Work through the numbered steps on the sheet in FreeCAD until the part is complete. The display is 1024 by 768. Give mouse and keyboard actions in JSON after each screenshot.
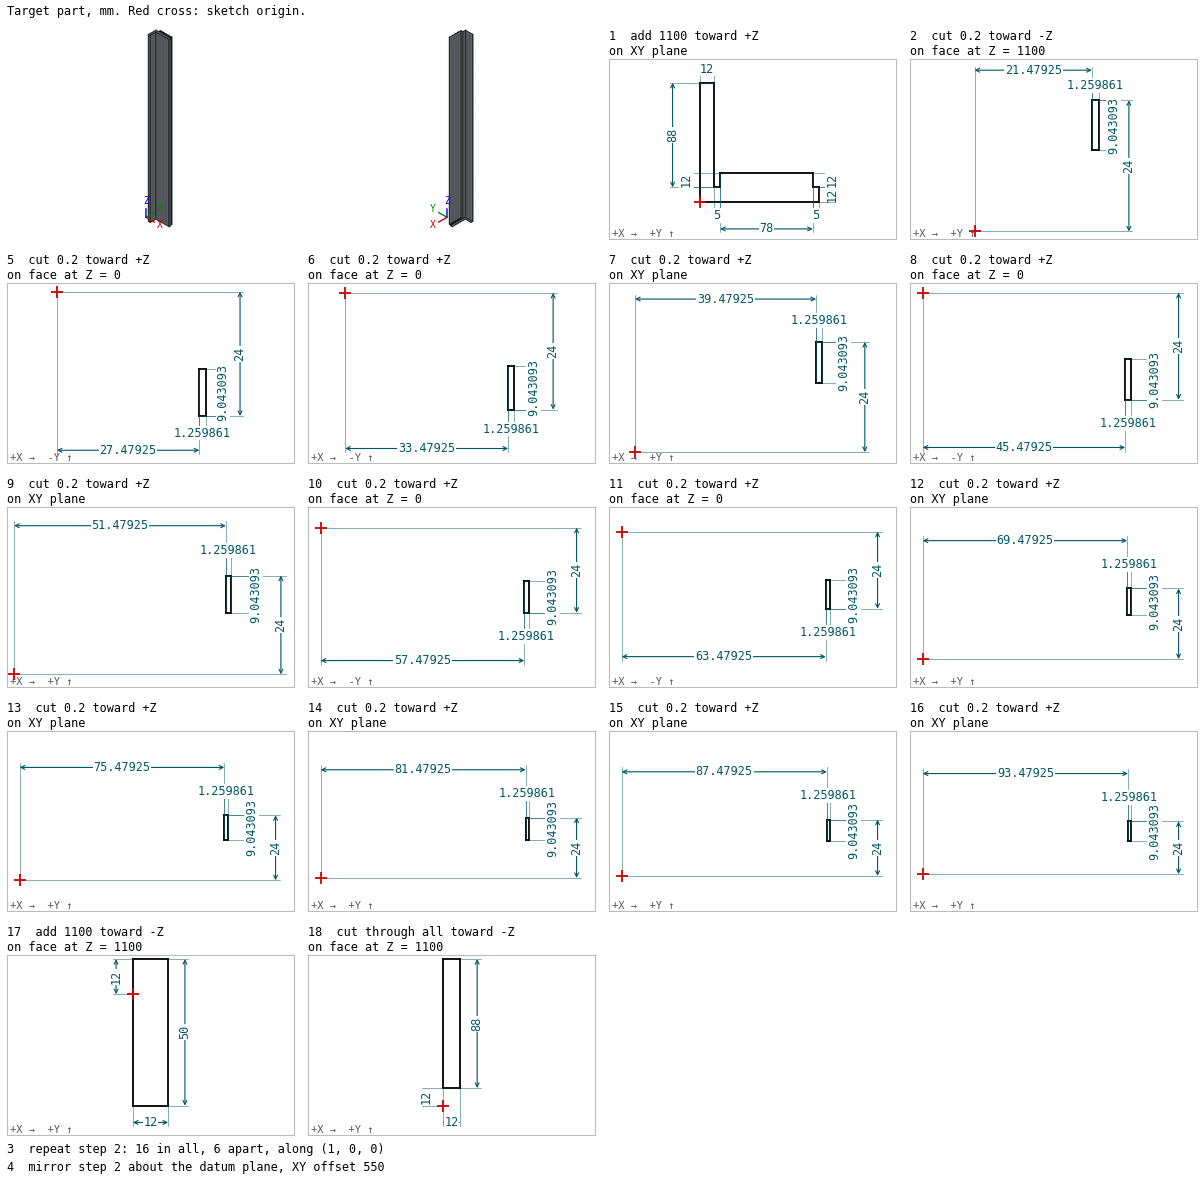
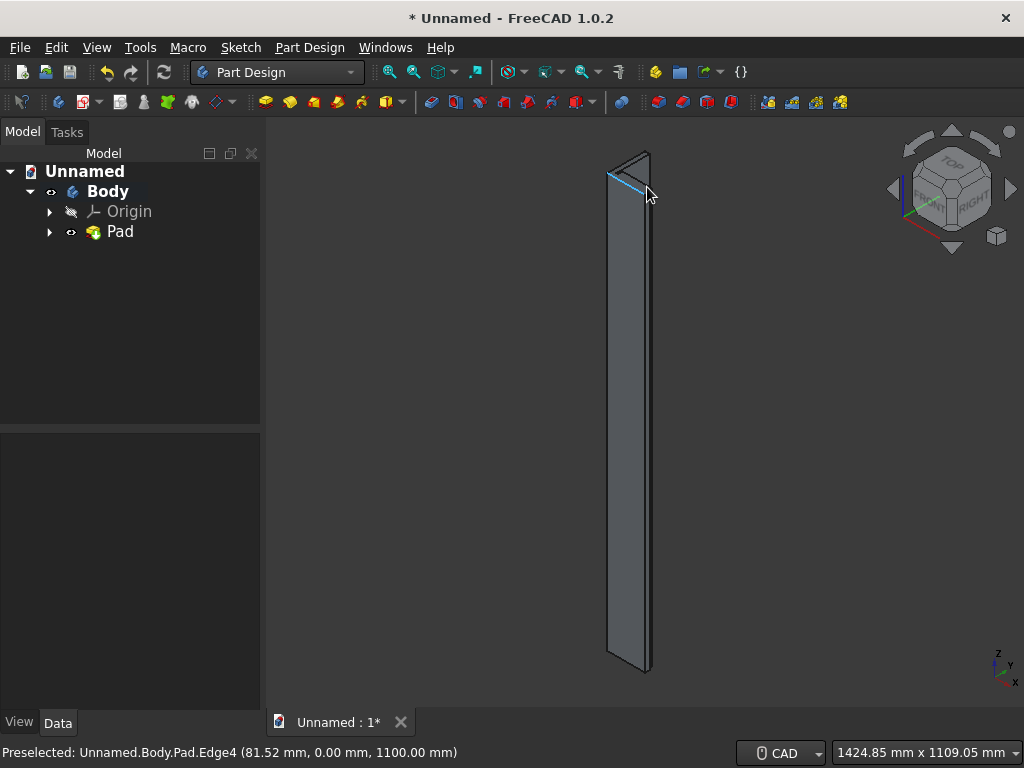
{"action": "scroll", "coordinate": [640, 188], "scroll_direction": "up", "scroll_amount": 6}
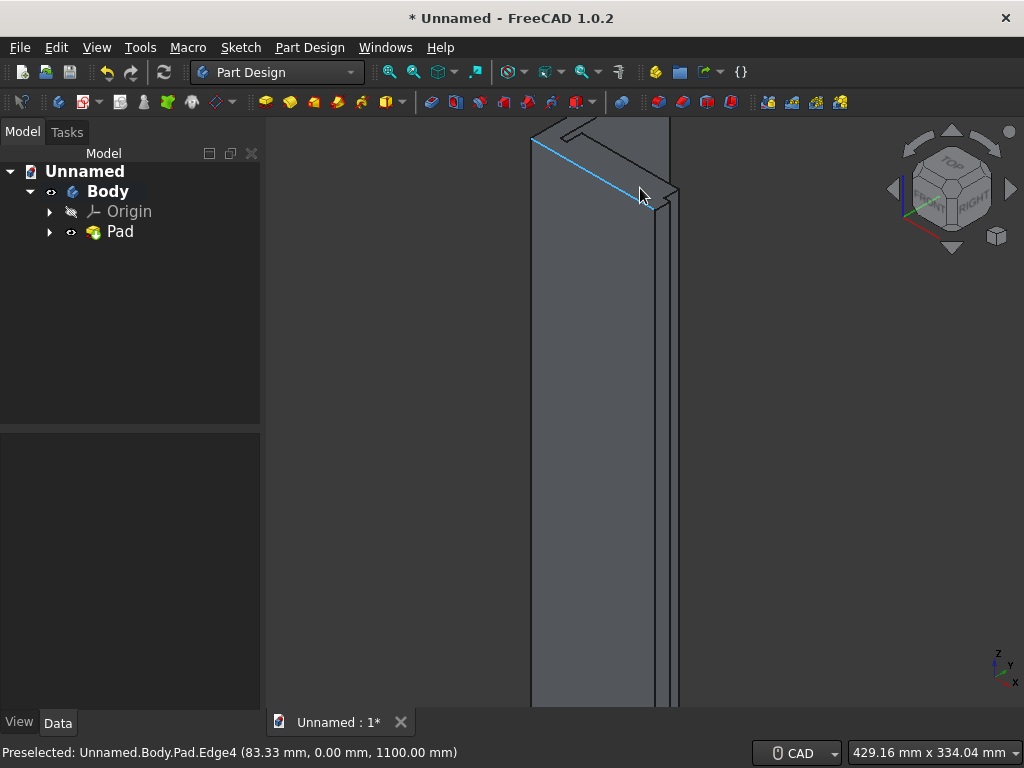
{"action": "left_click", "coordinate": [620, 178]}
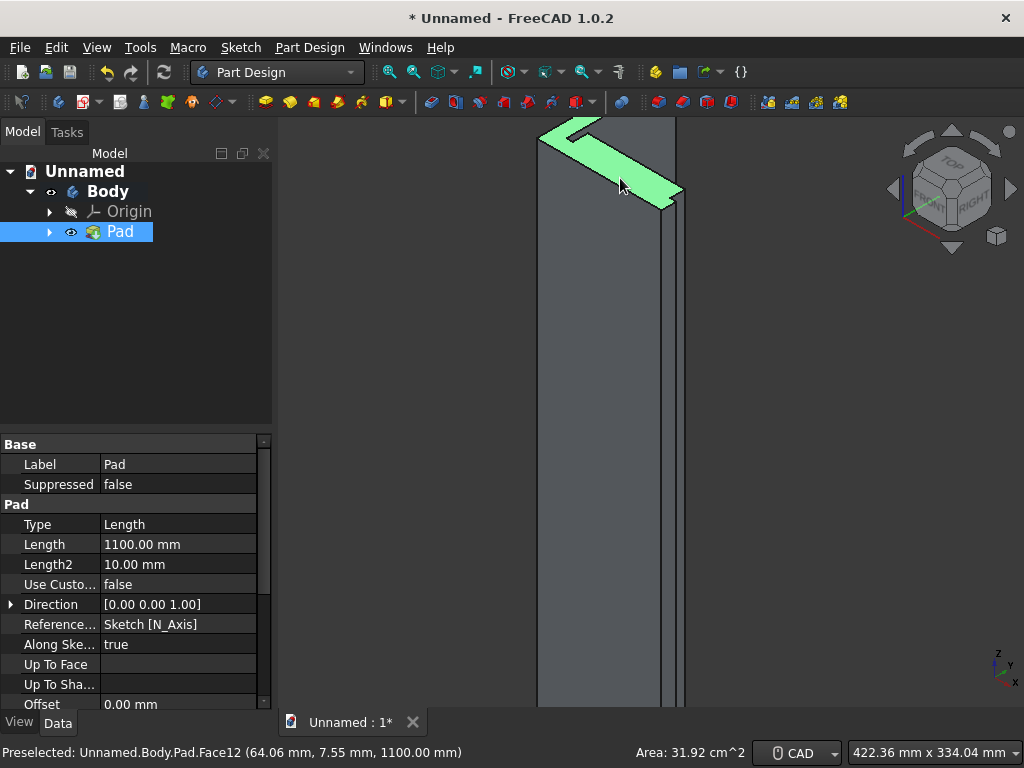
{"action": "left_click", "coordinate": [84, 102]}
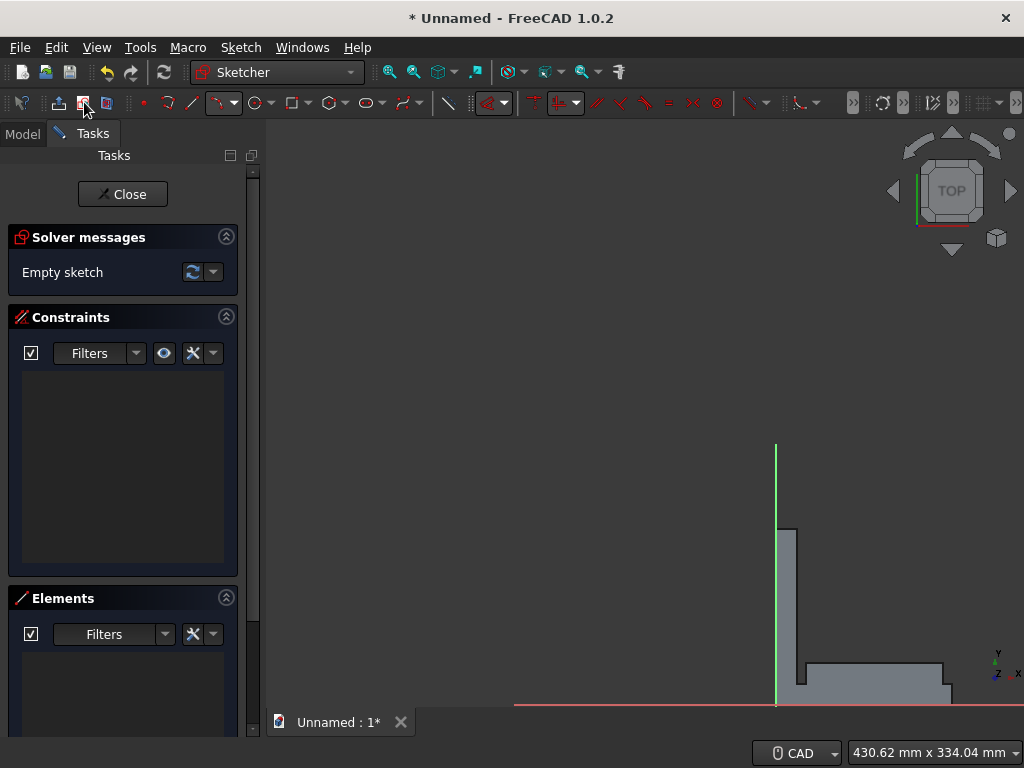
{"action": "scroll", "coordinate": [576, 413], "scroll_direction": "down", "scroll_amount": 5}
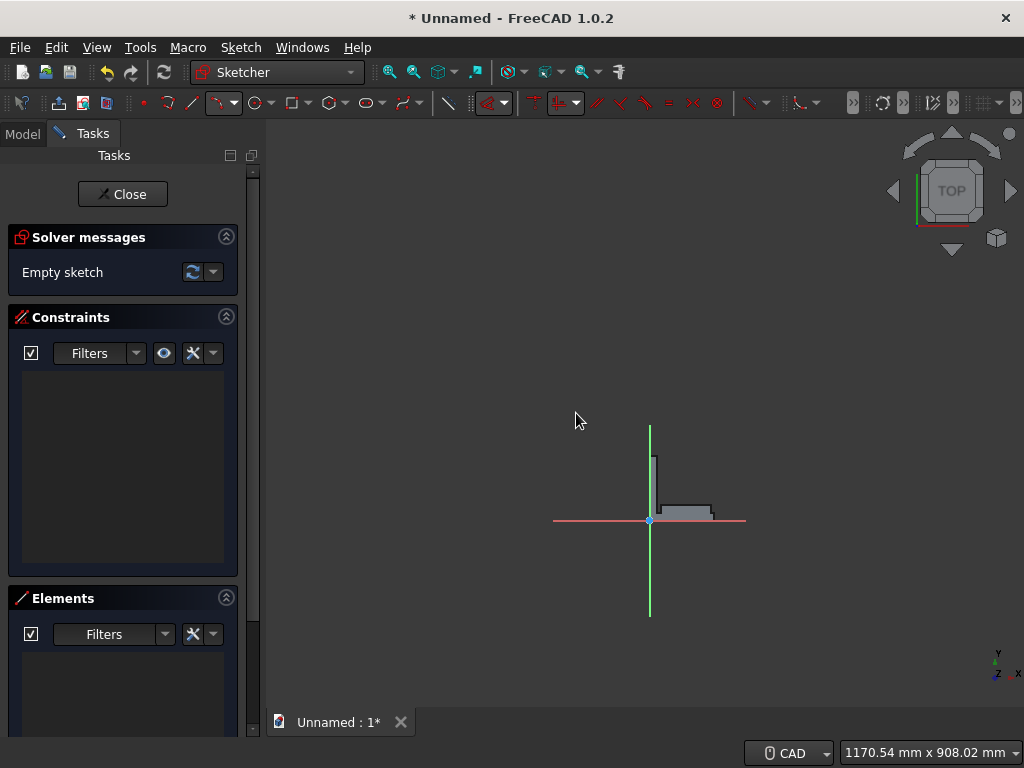
{"action": "scroll", "coordinate": [669, 513], "scroll_direction": "up", "scroll_amount": 15}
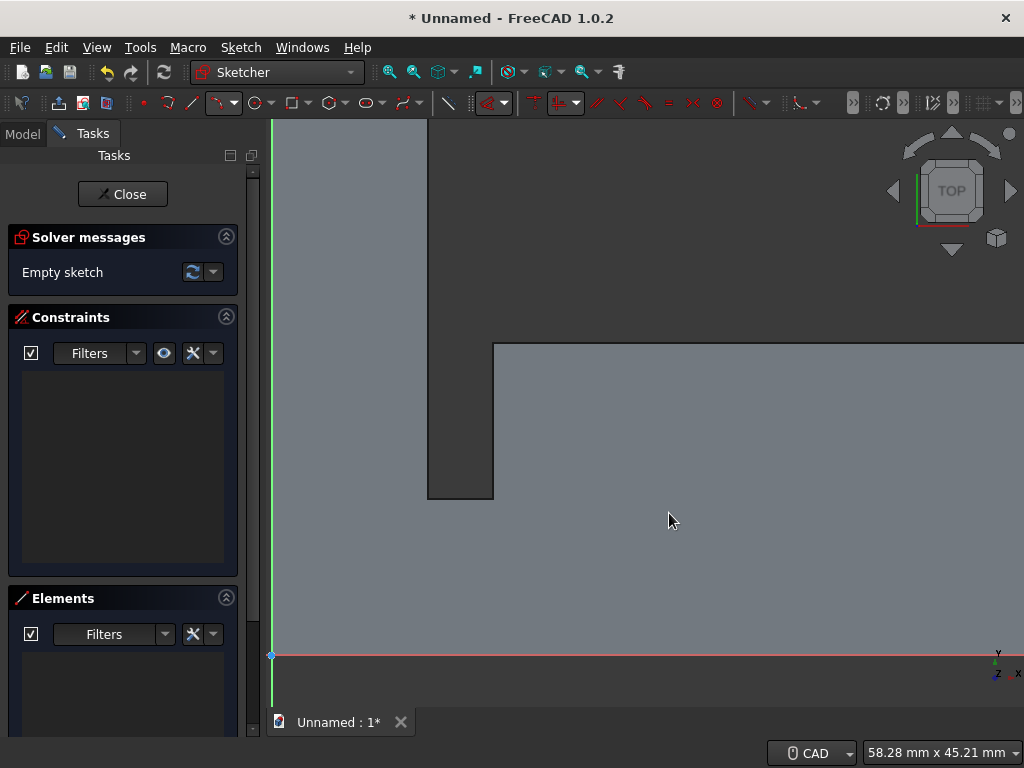
{"action": "scroll", "coordinate": [552, 397], "scroll_direction": "up", "scroll_amount": 6}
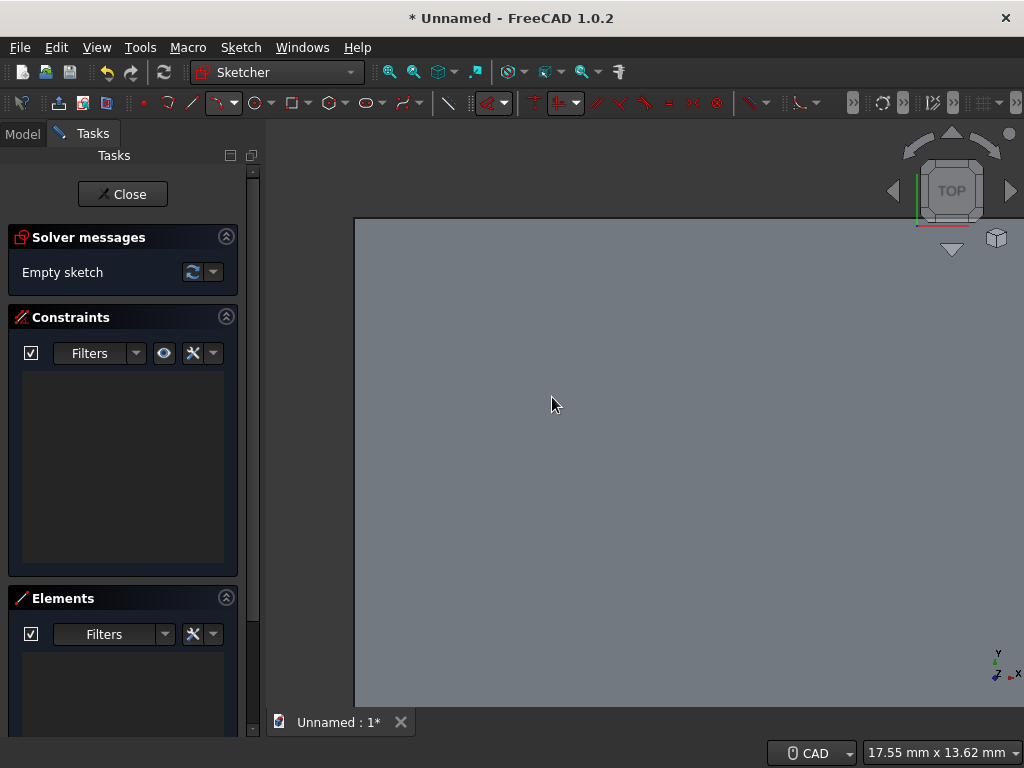
{"action": "left_click", "coordinate": [292, 104]}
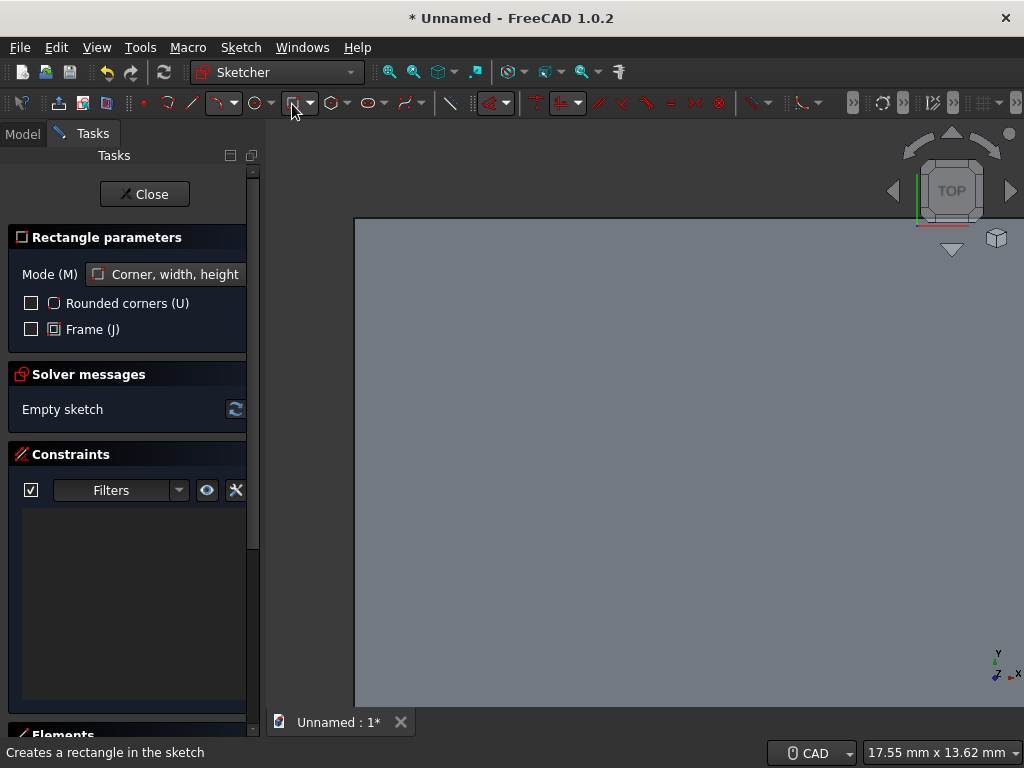
{"action": "left_click", "coordinate": [548, 218]}
{"action": "mouse_move", "coordinate": [602, 608]}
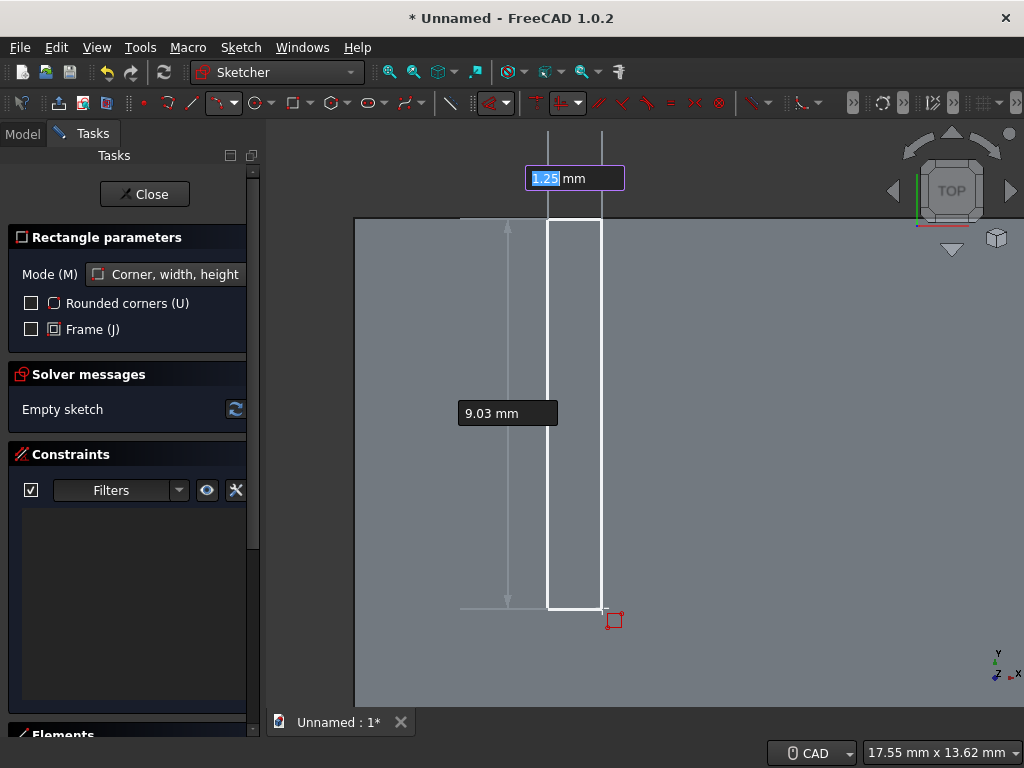
{"action": "type", "text": "1.259861"}
{"action": "key", "text": "Tab"}
{"action": "type", "text": "9.043093"}
{"action": "key", "text": "Return"}
{"action": "key", "text": "Escape"}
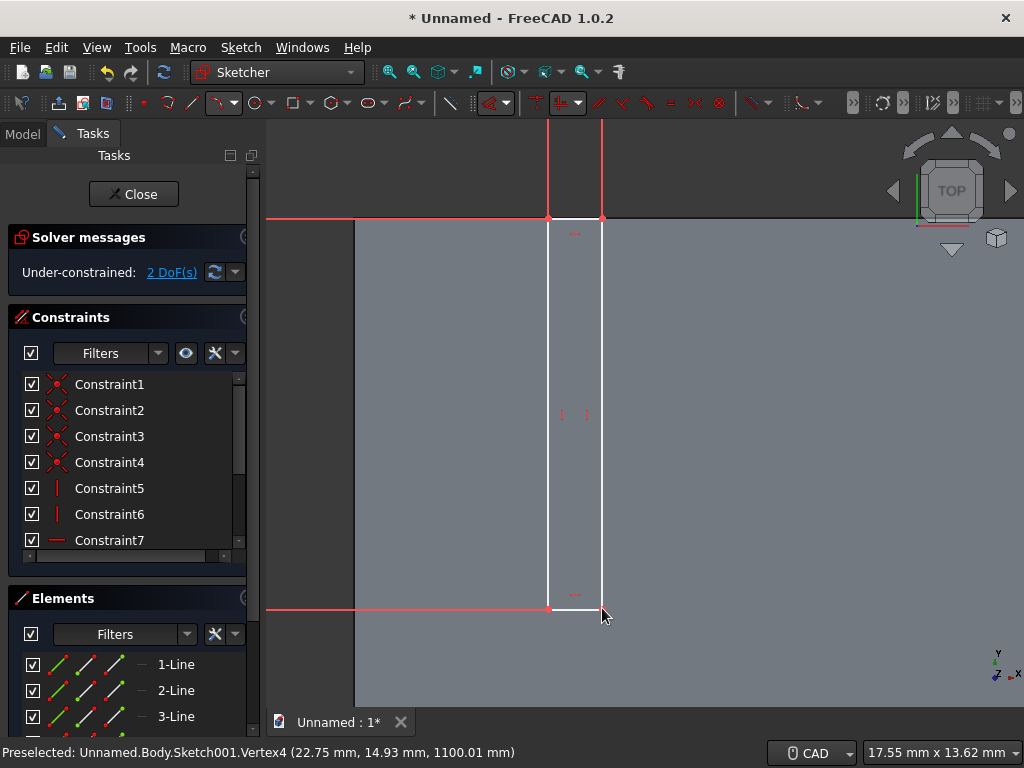
{"action": "left_click", "coordinate": [548, 219]}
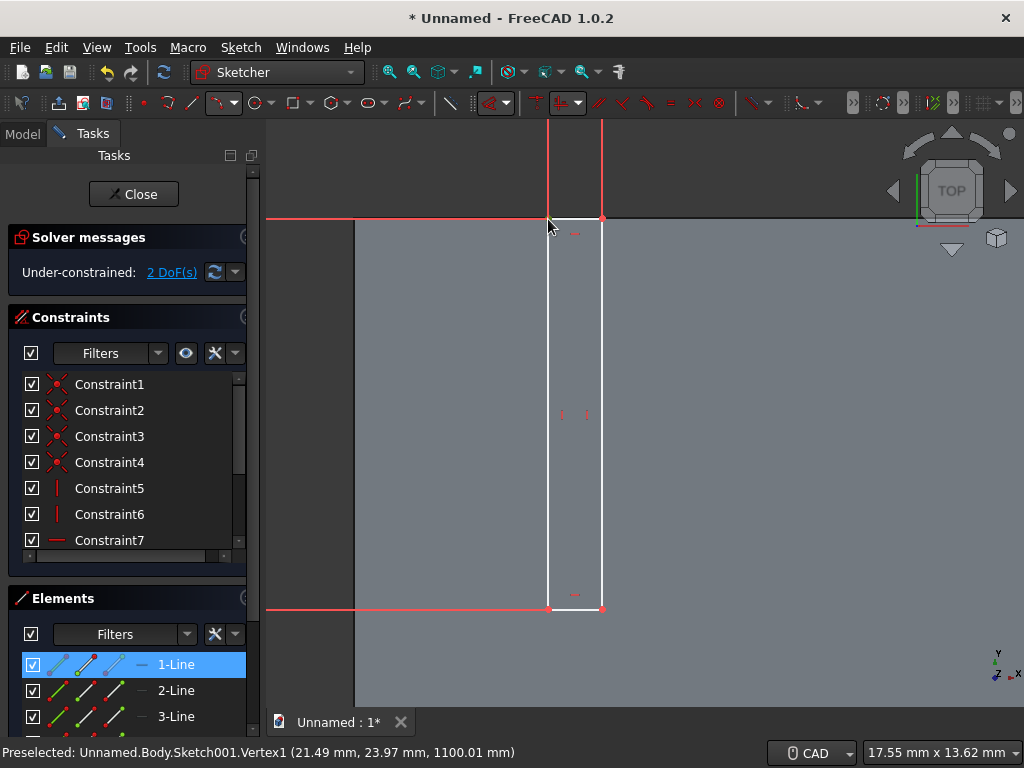
{"action": "left_click", "coordinate": [508, 104]}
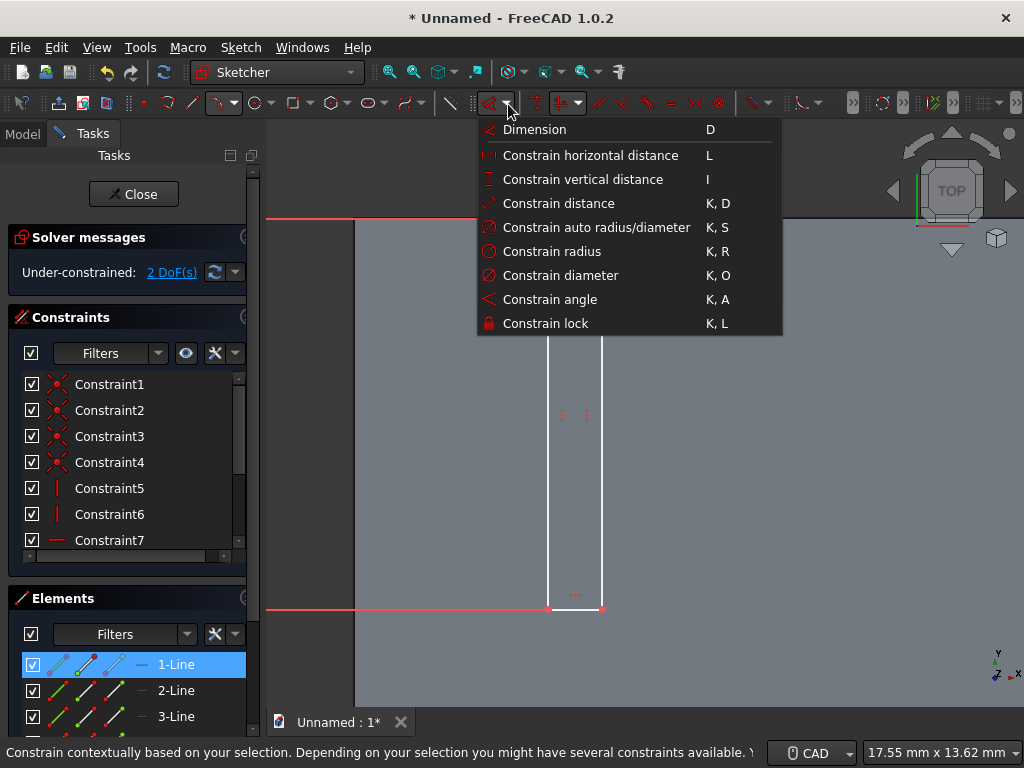
{"action": "left_click", "coordinate": [630, 179]}